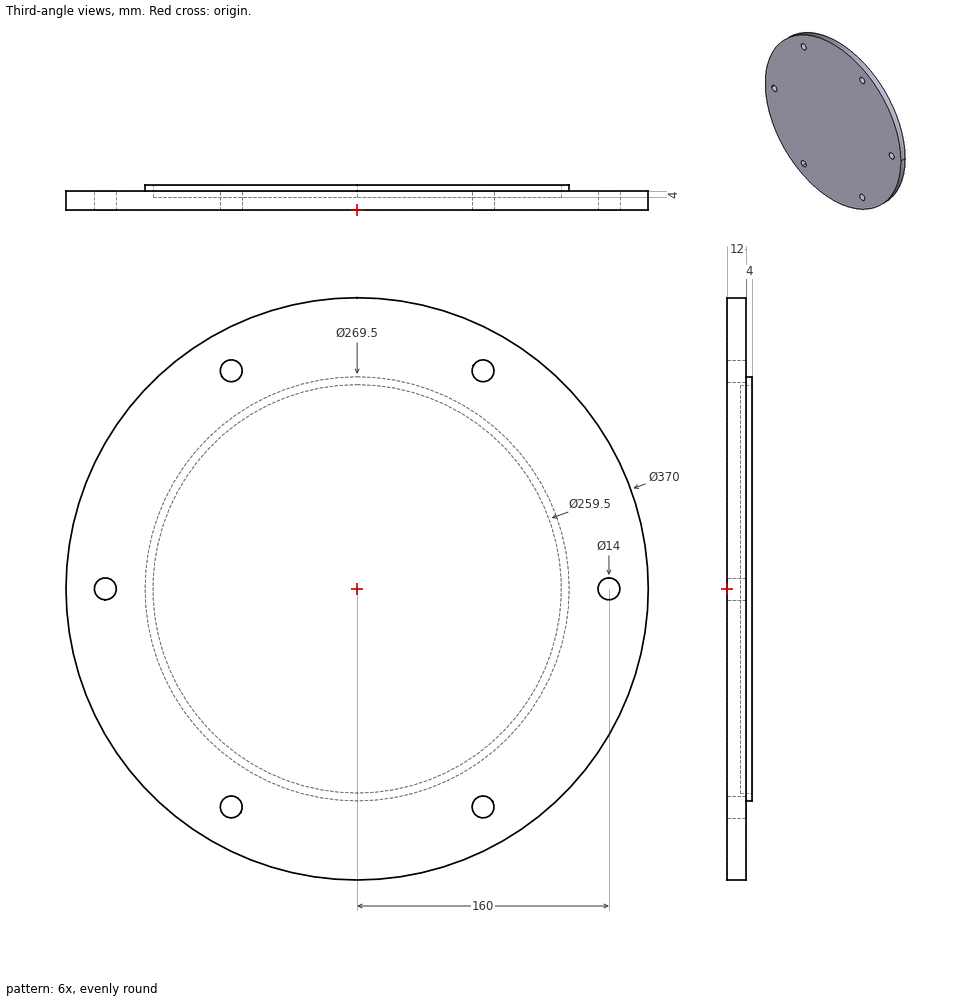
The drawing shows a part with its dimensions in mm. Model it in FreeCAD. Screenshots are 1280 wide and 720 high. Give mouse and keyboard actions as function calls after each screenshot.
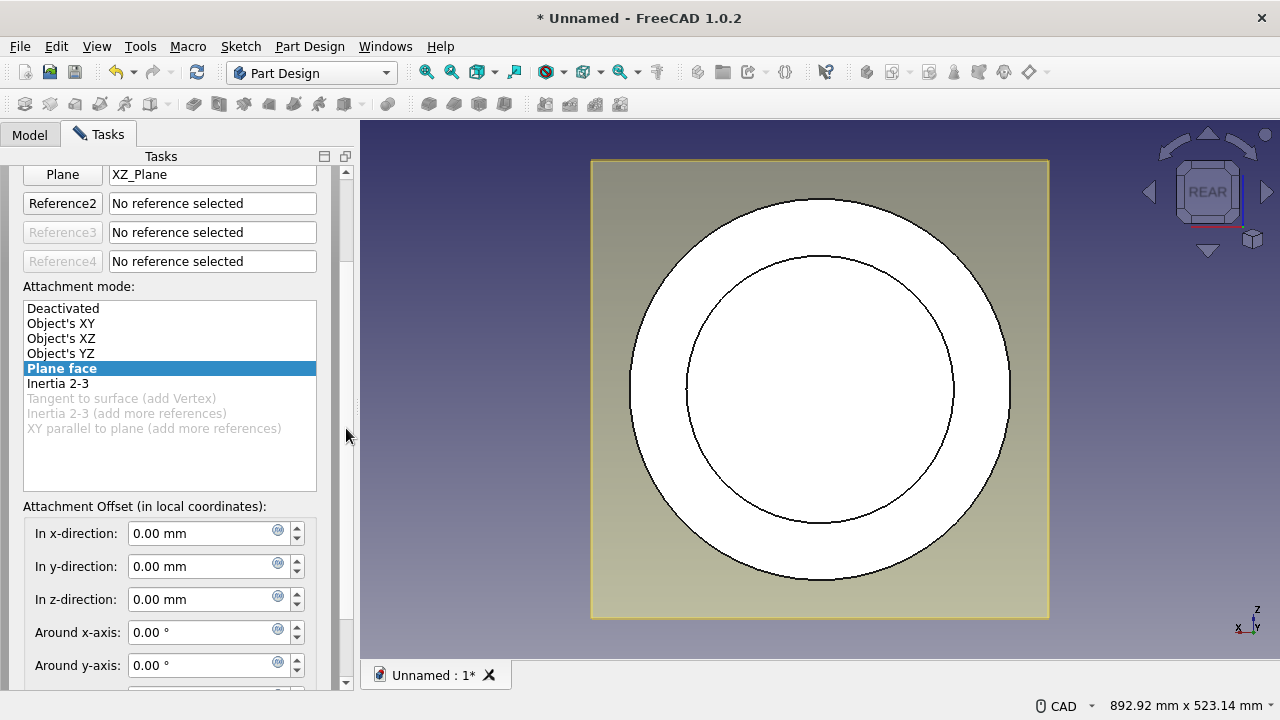
triple_click(210, 600)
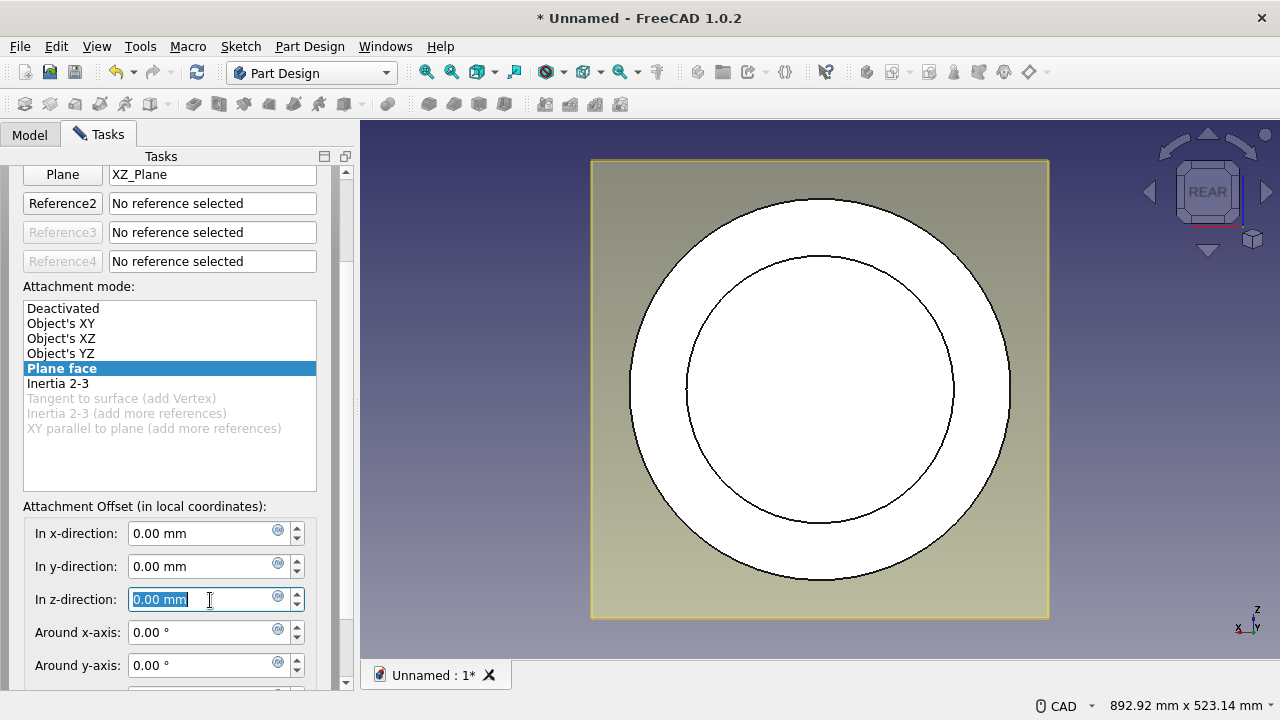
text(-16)
key(Tab)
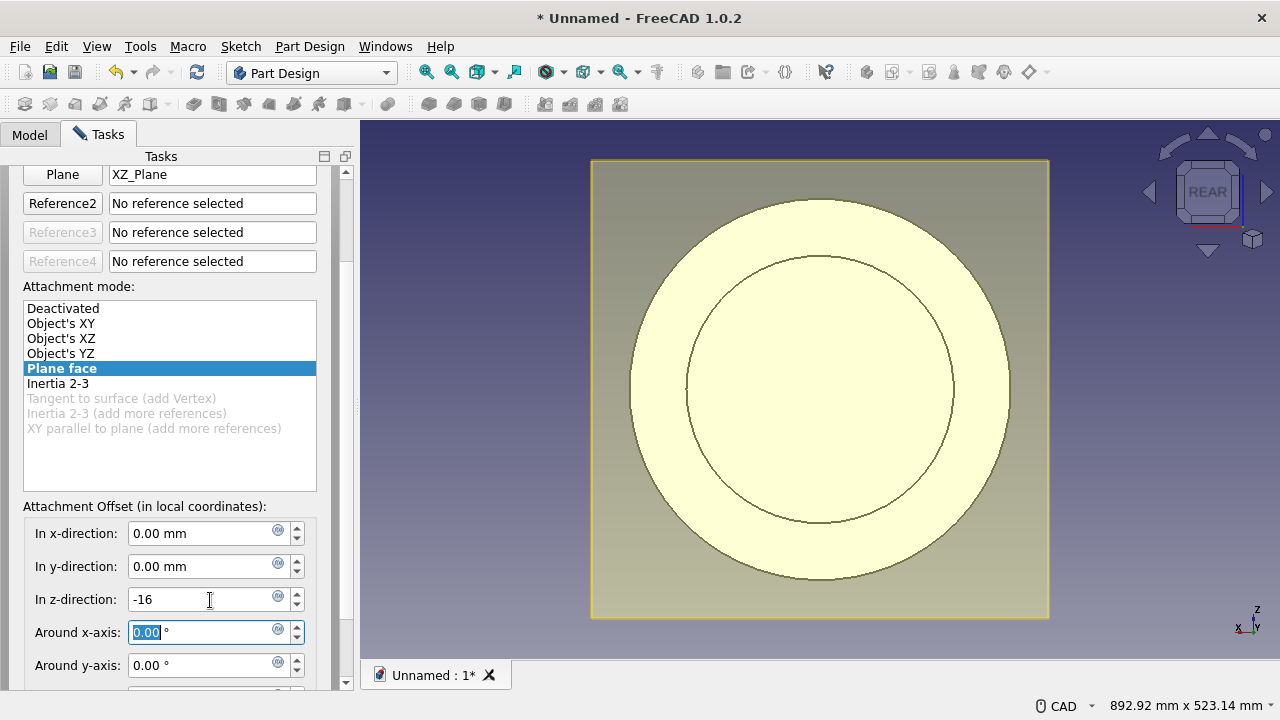
scroll(346, 428, up, 3)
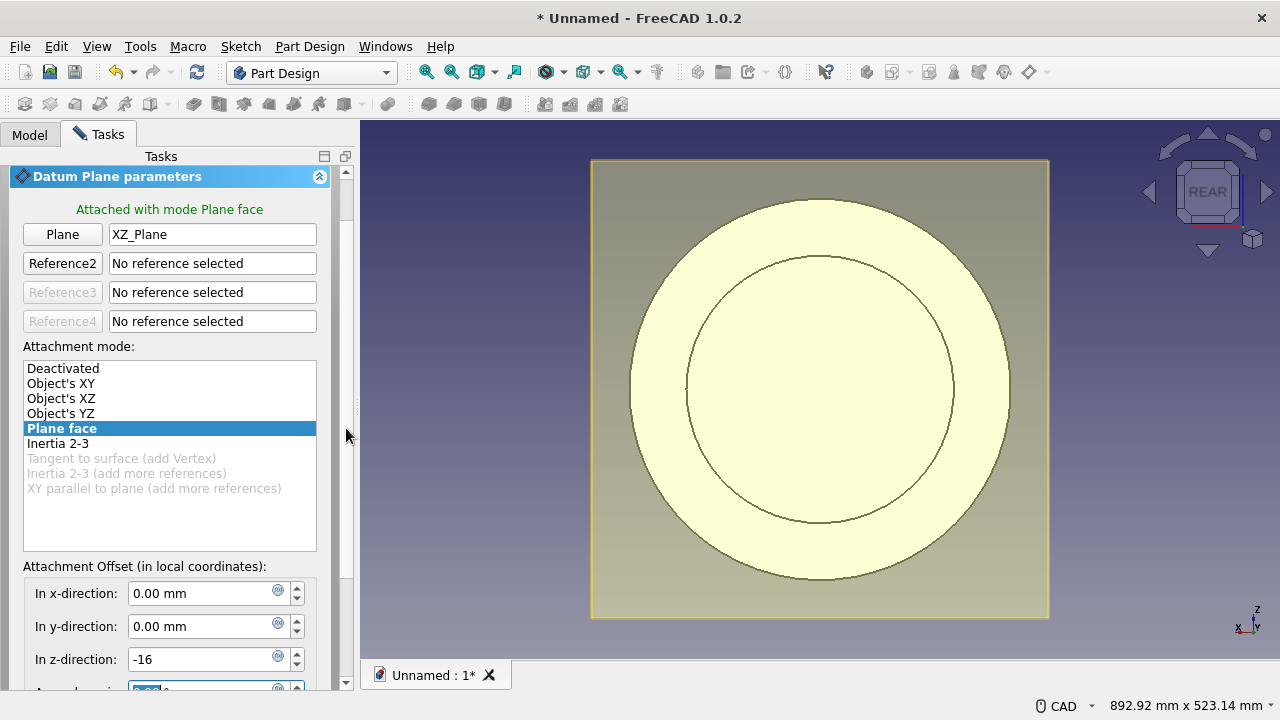
click(127, 195)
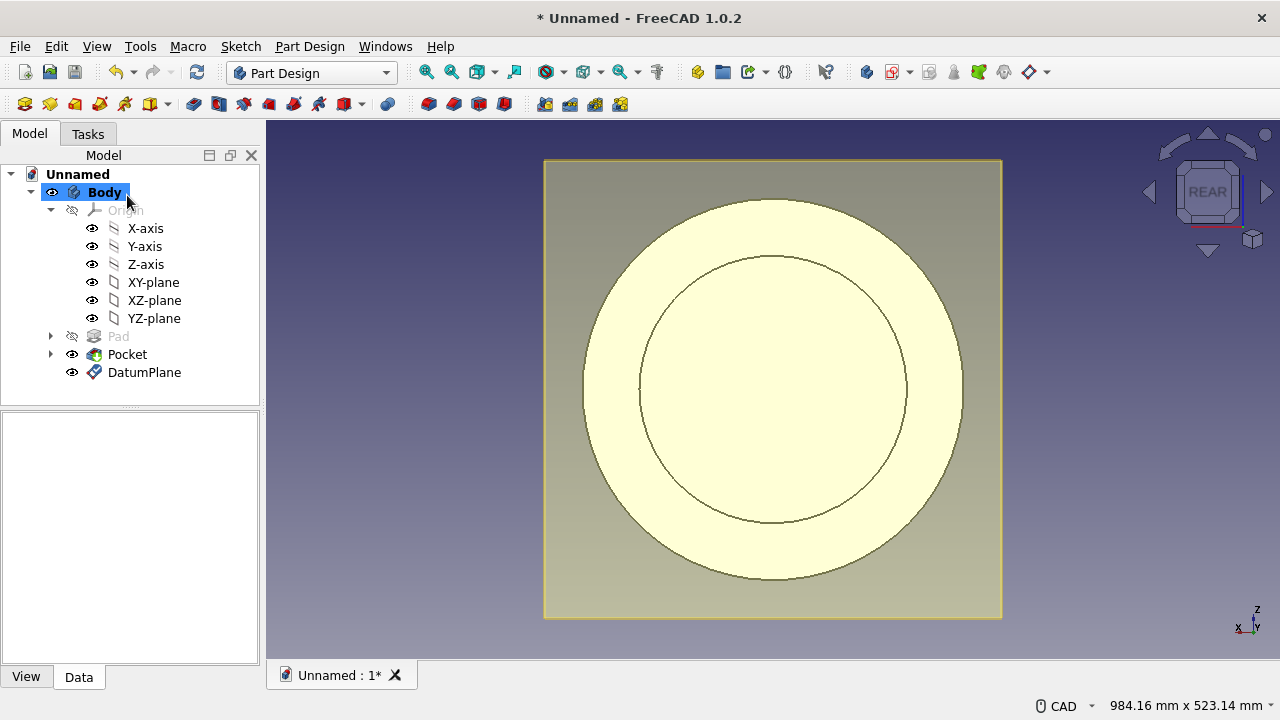
click(117, 372)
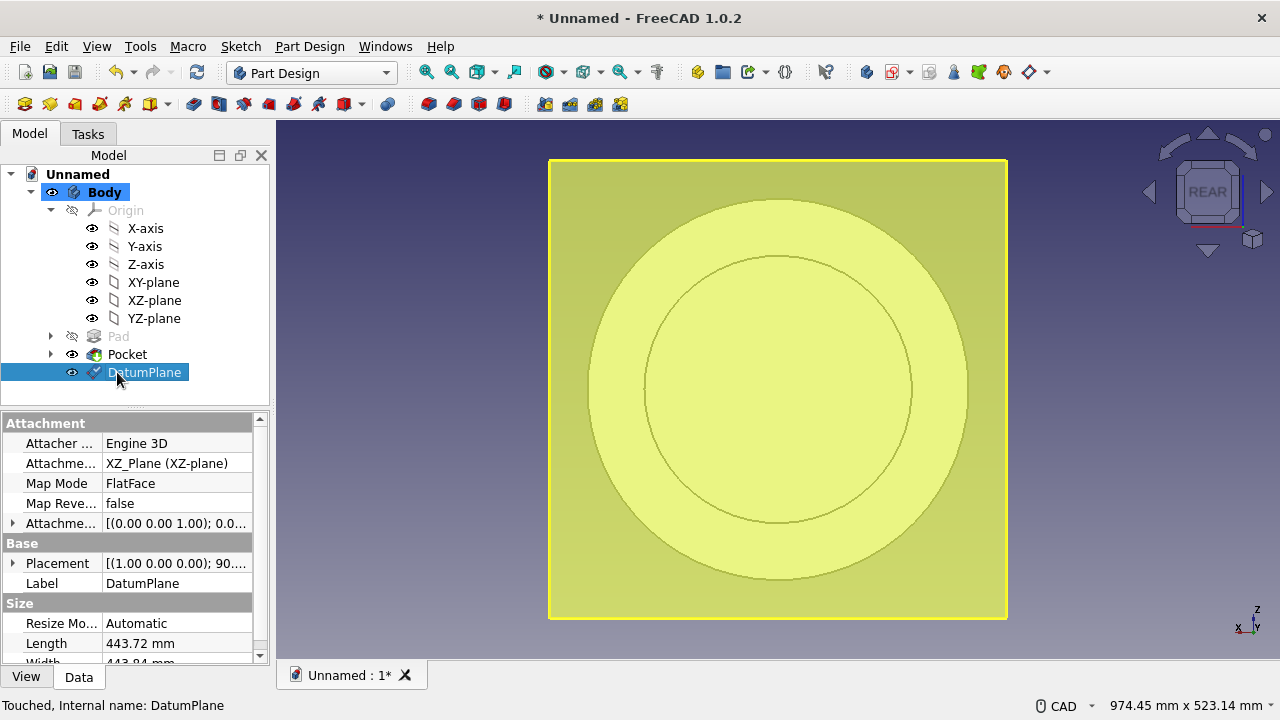
click(892, 72)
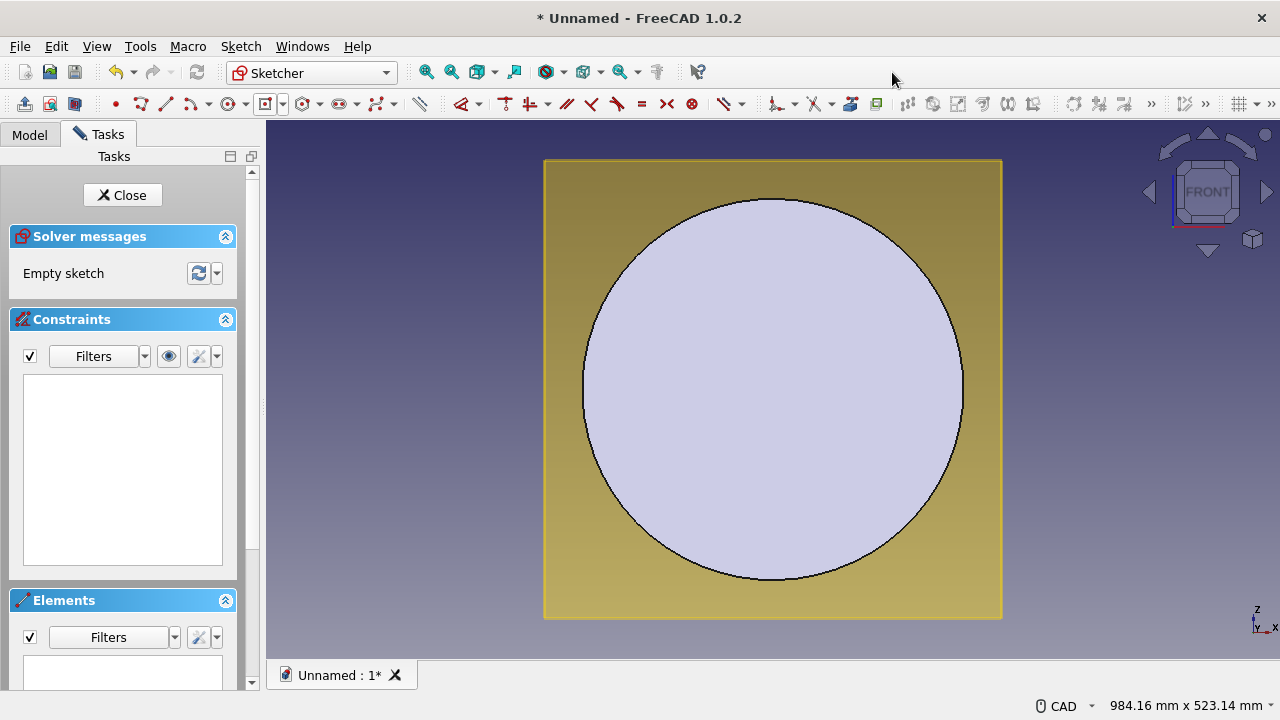
click(75, 104)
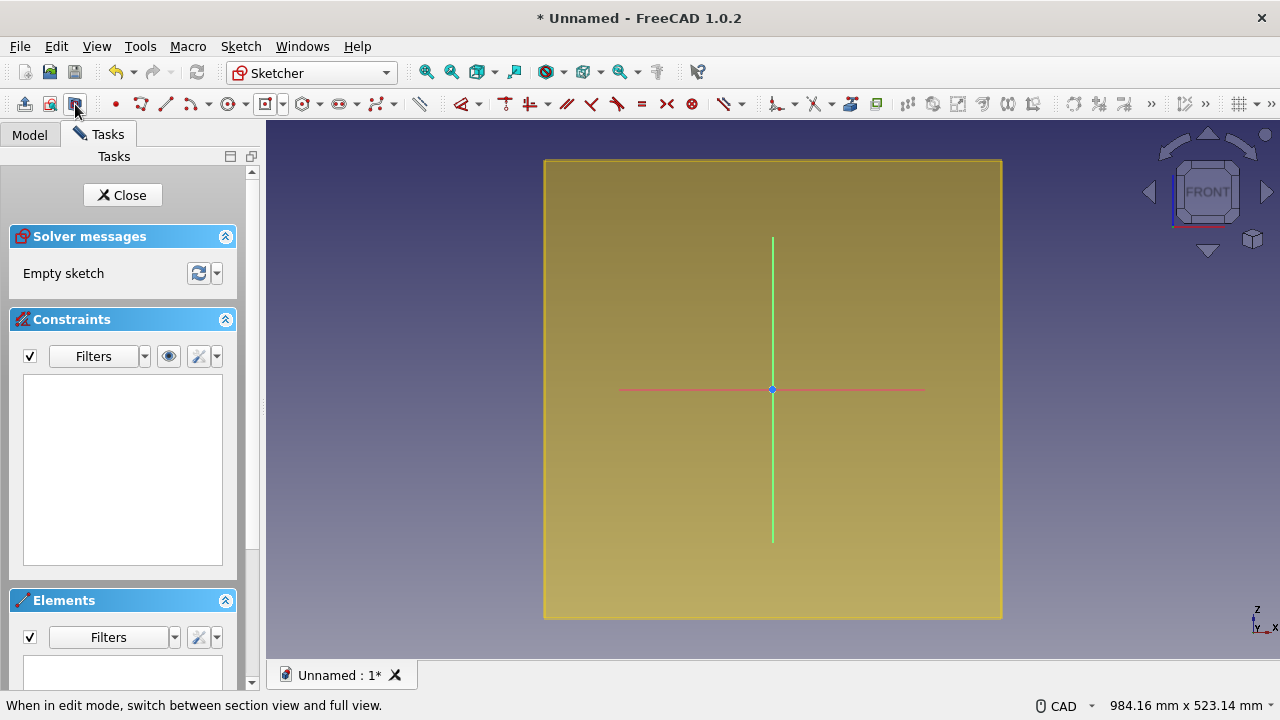
click(228, 104)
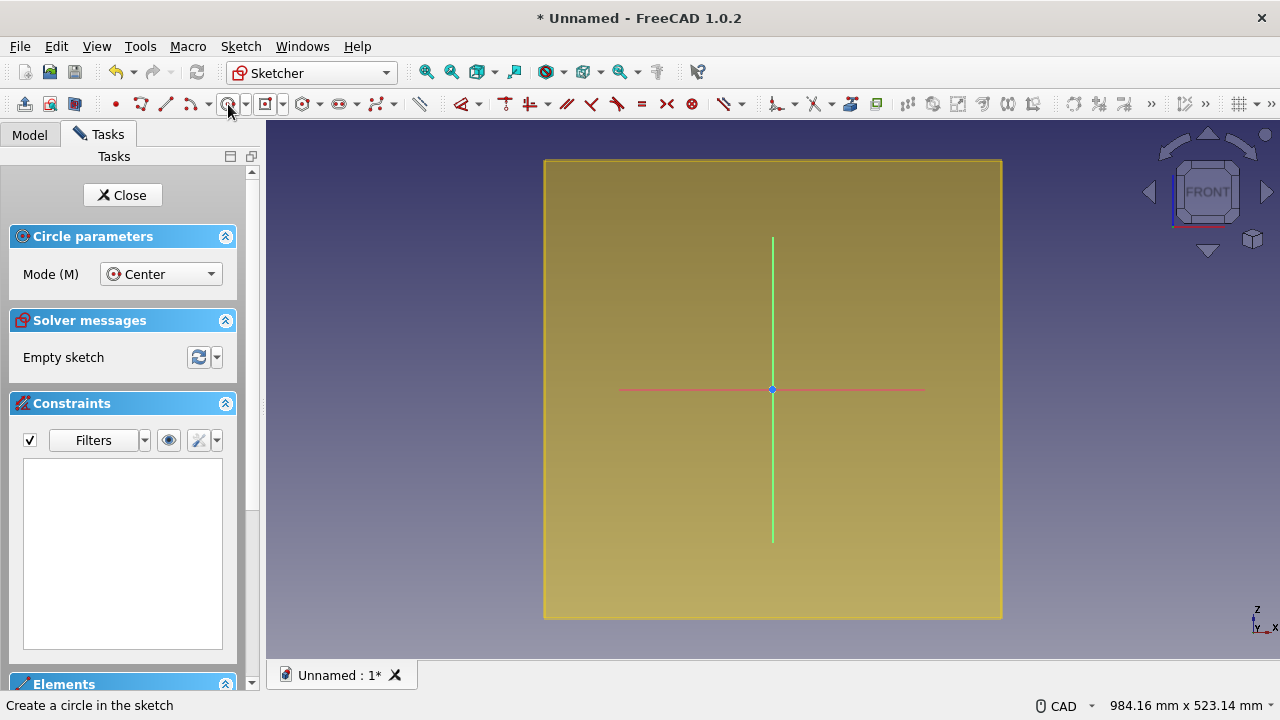
click(773, 390)
click(871, 291)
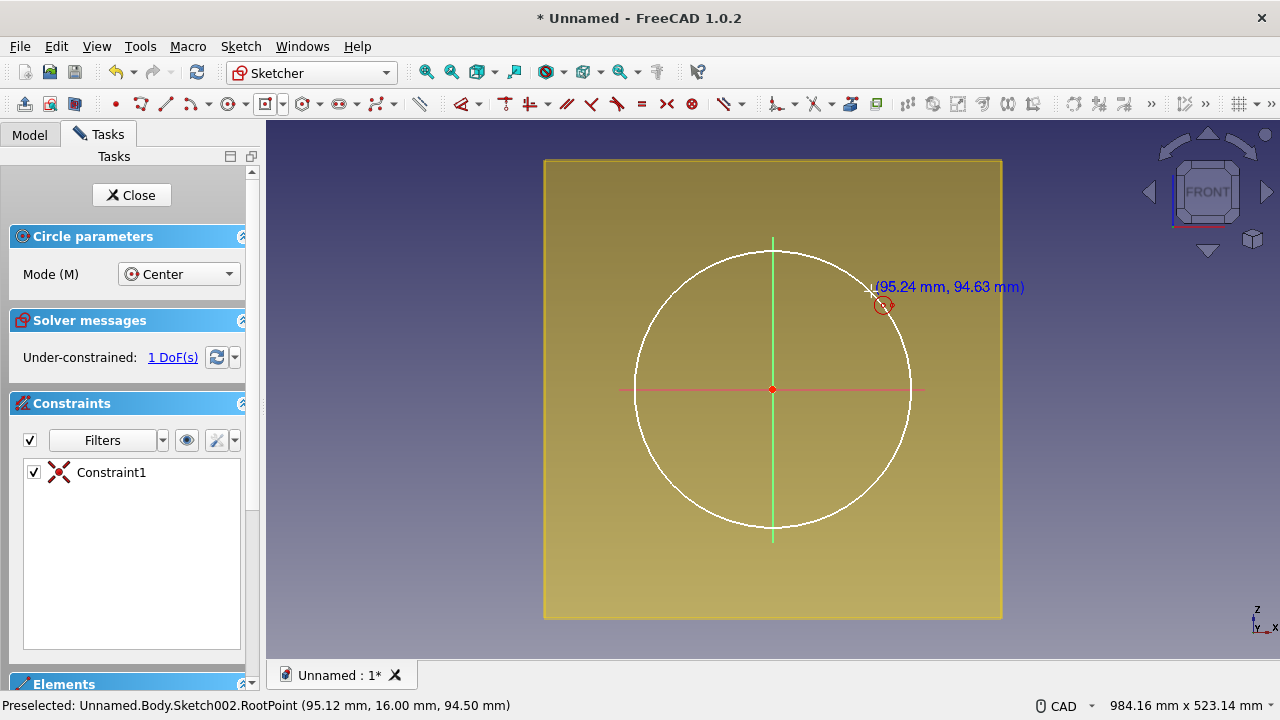
click(773, 390)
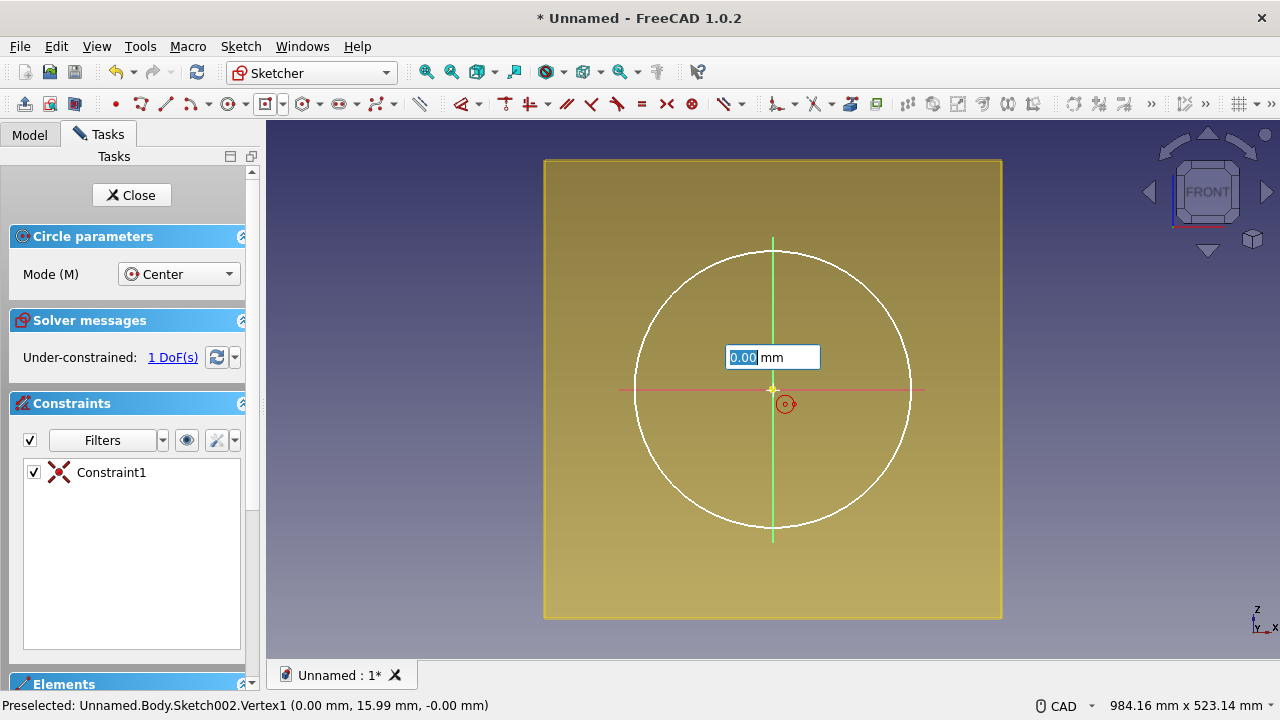
scroll(867, 295, up, 6)